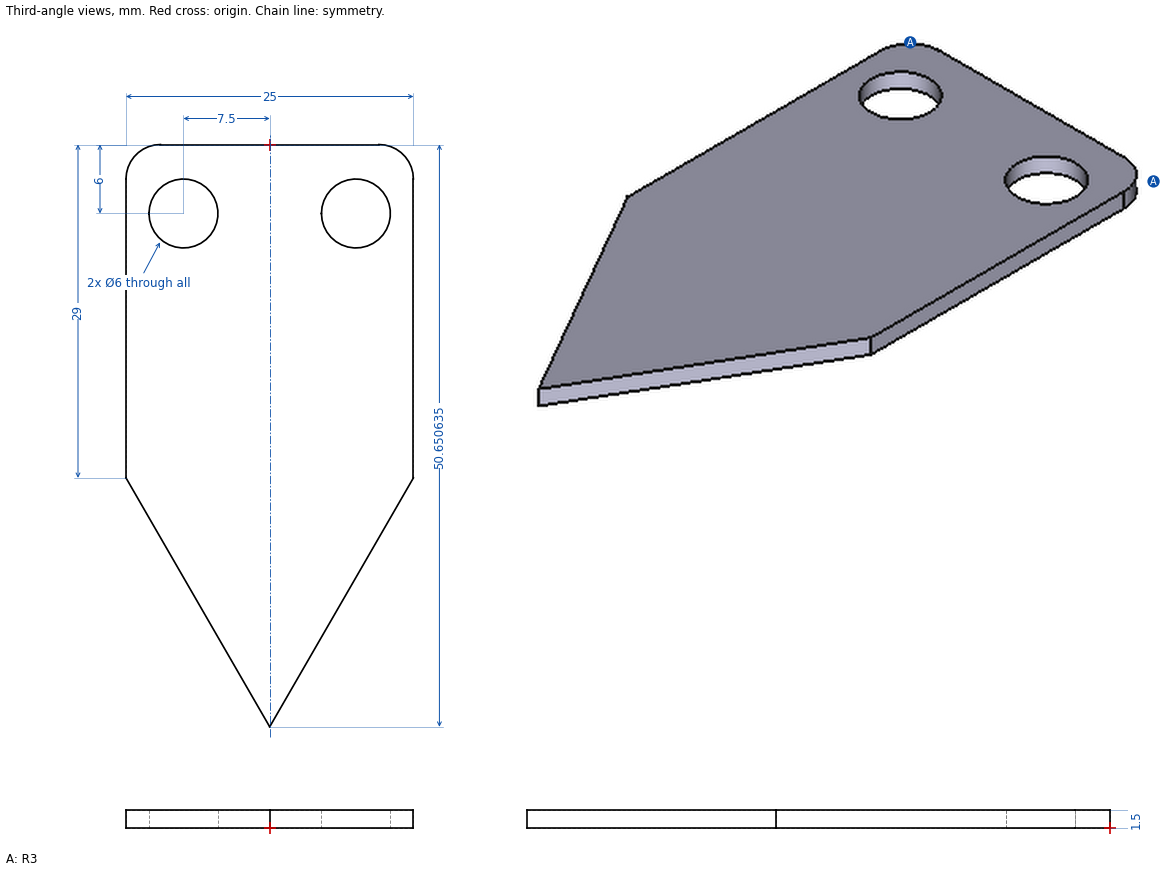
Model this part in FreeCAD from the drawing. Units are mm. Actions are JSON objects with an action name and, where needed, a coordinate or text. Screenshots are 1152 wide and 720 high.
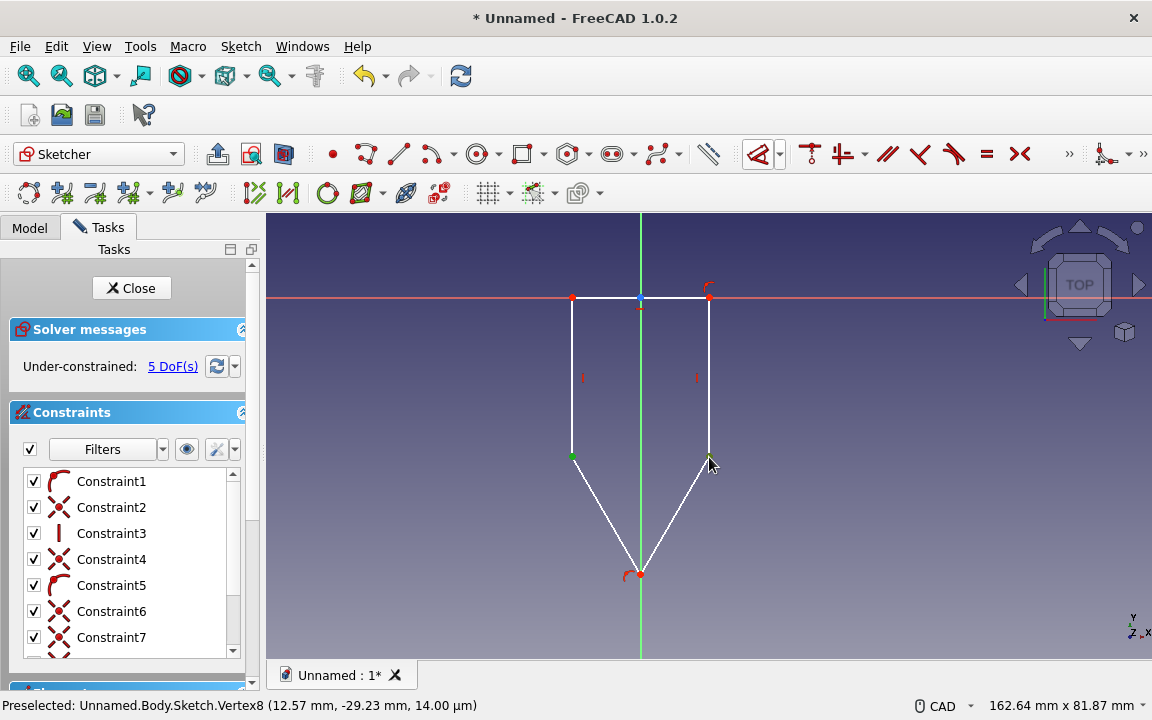
{"action": "left_click", "coordinate": [641, 492]}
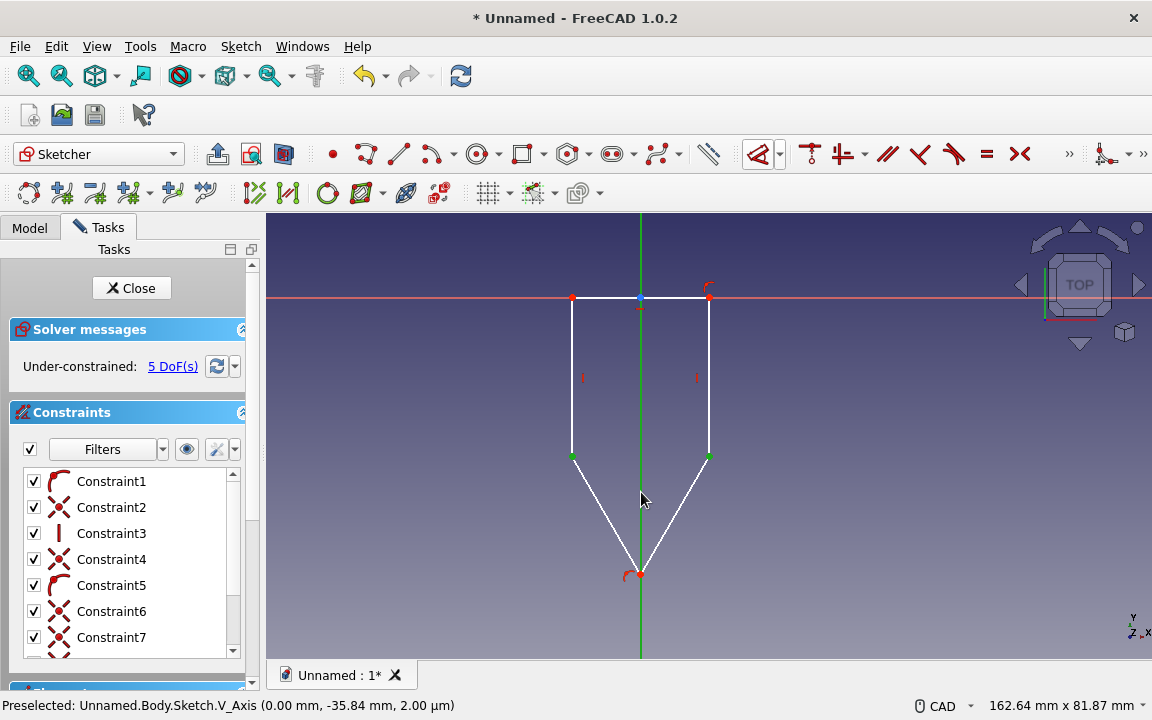
{"action": "left_click", "coordinate": [1020, 154]}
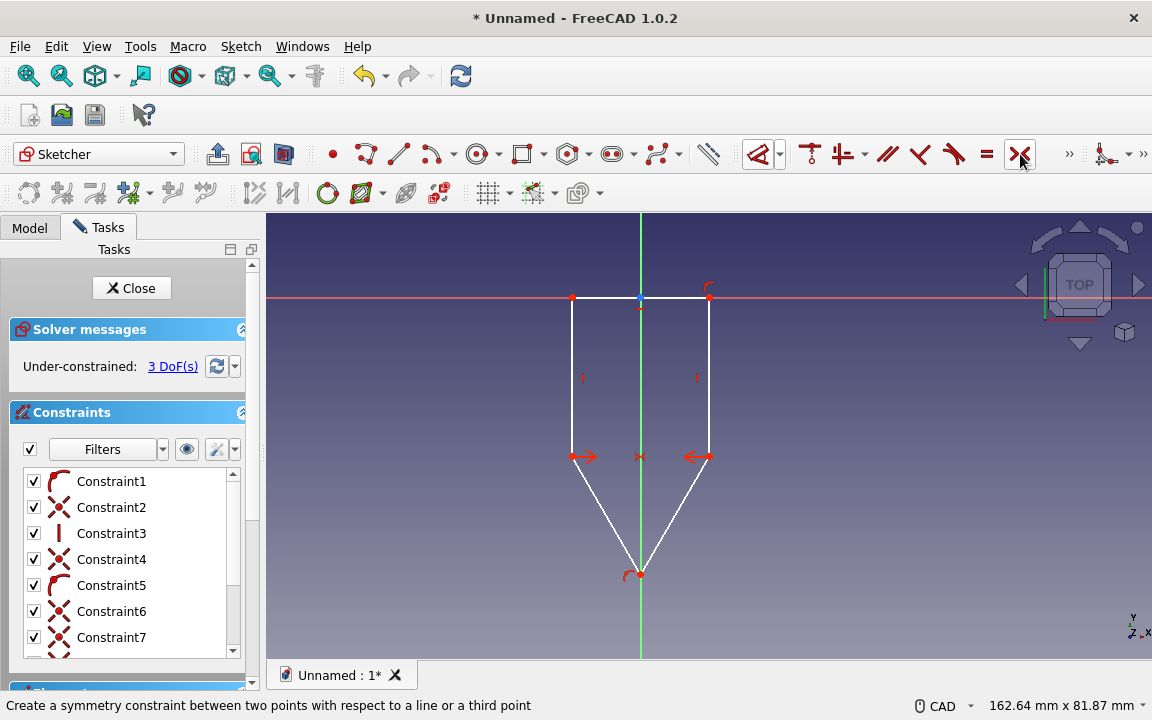
{"action": "left_click", "coordinate": [758, 154]}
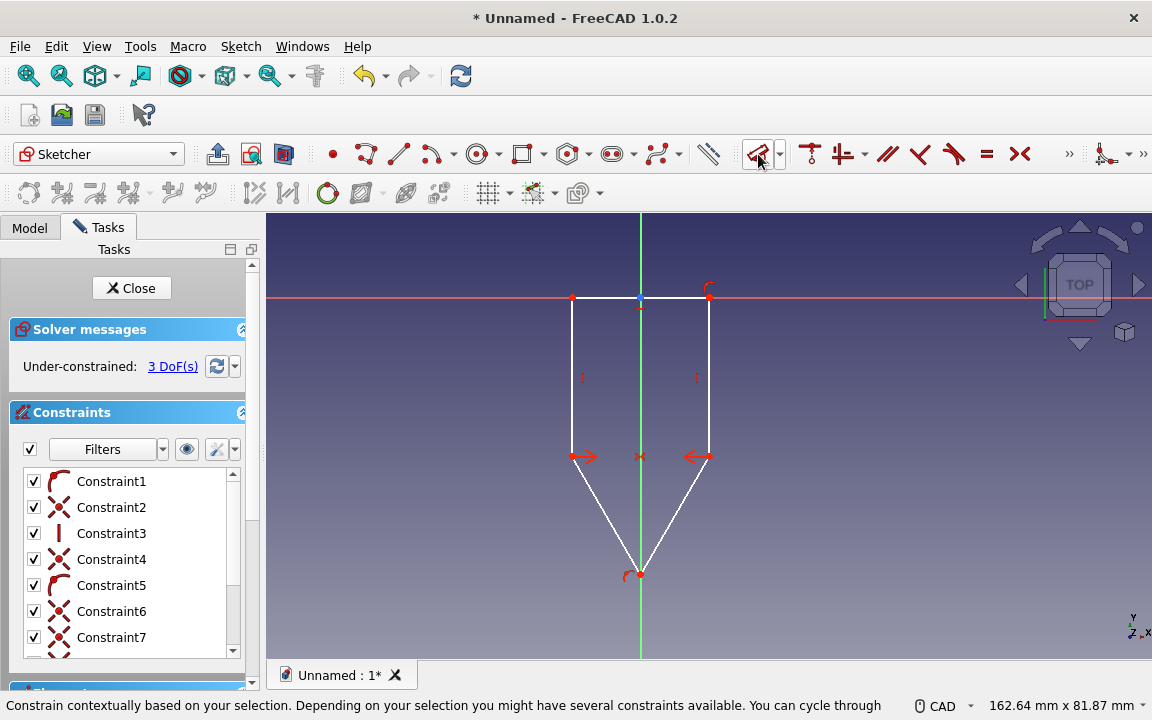
{"action": "left_click", "coordinate": [668, 298]}
{"action": "left_click", "coordinate": [609, 264]}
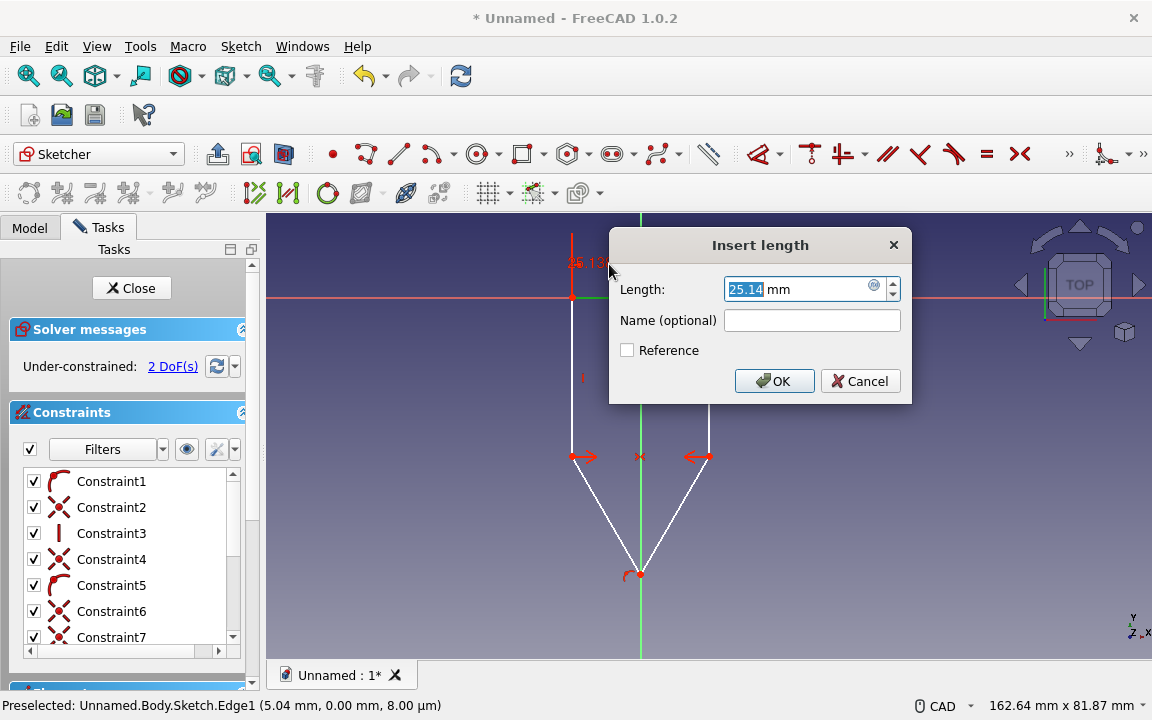
{"action": "type", "text": "25"}
{"action": "key", "text": "Return"}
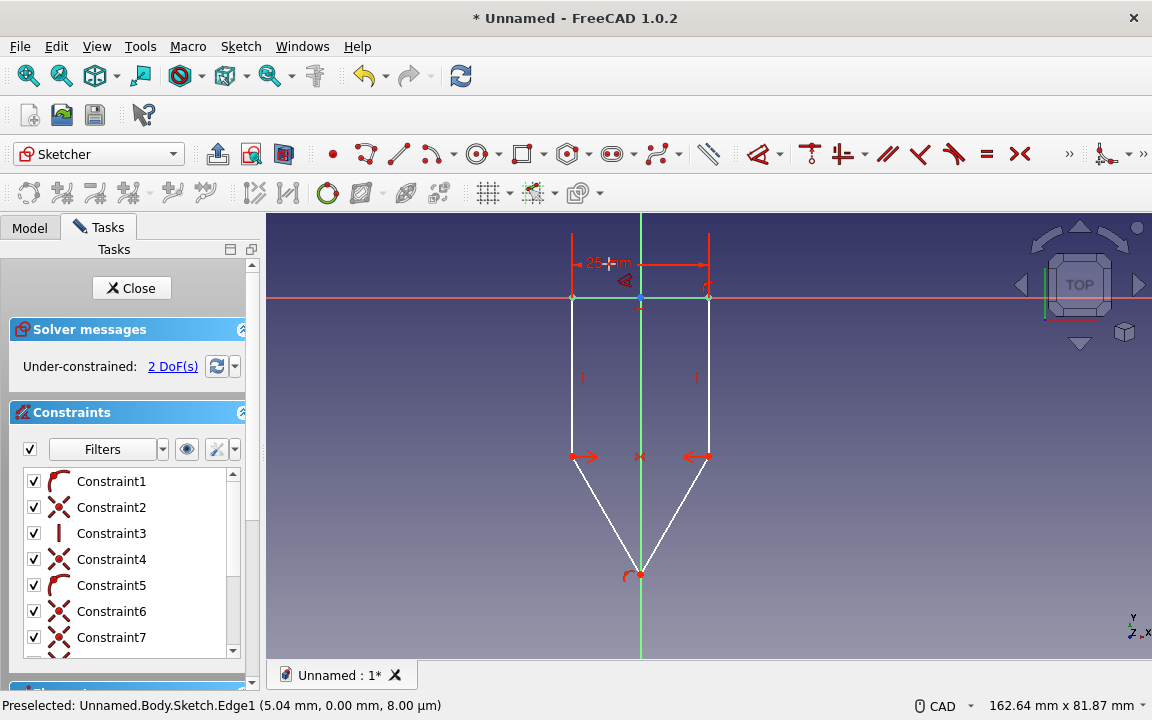
{"action": "left_click", "coordinate": [572, 346]}
{"action": "left_click", "coordinate": [538, 377]}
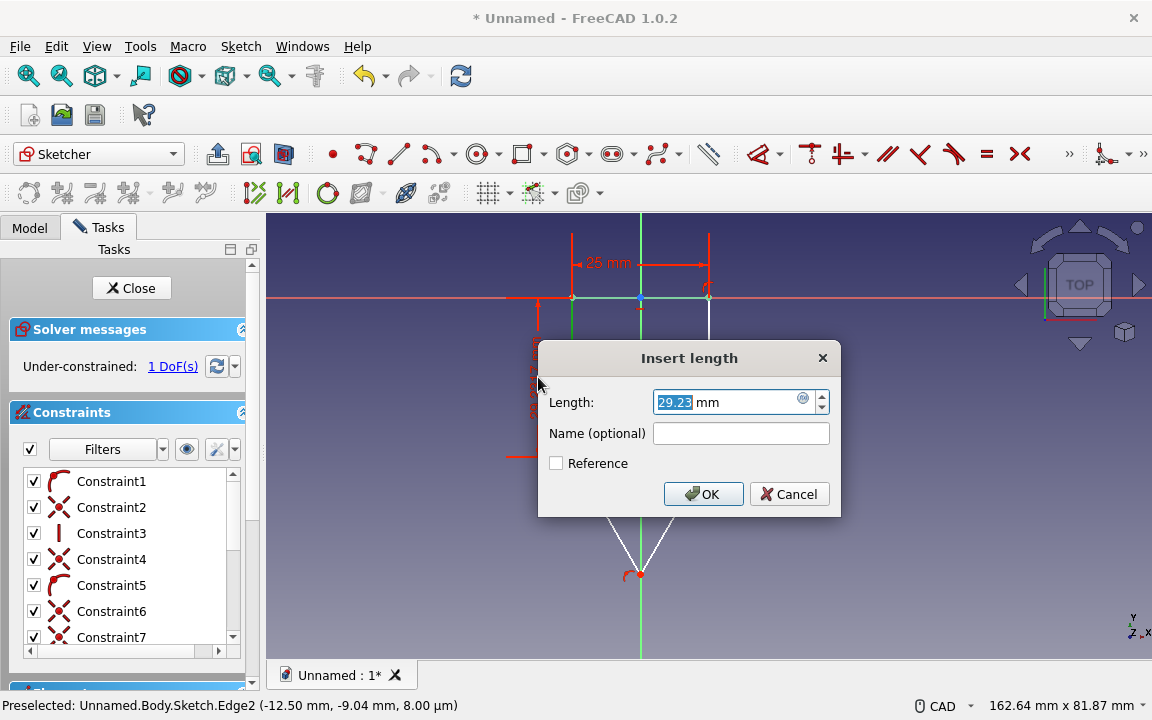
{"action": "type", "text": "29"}
{"action": "key", "text": "Return"}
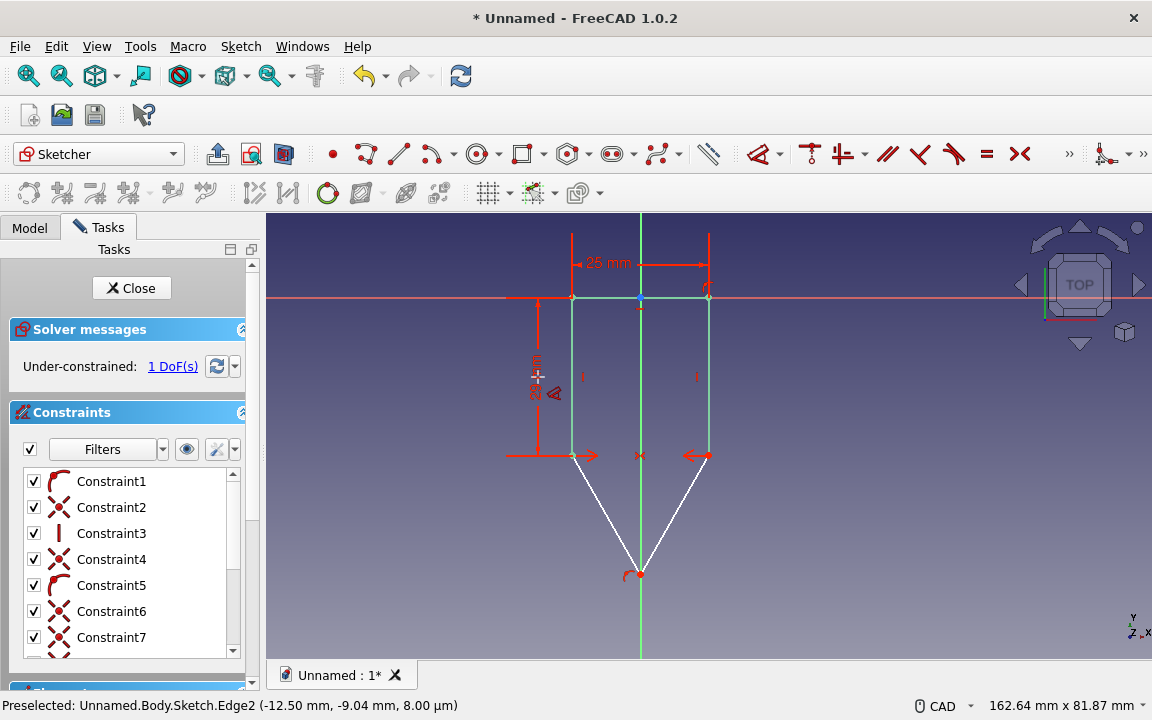
{"action": "left_click", "coordinate": [641, 575]}
{"action": "left_click", "coordinate": [675, 436]}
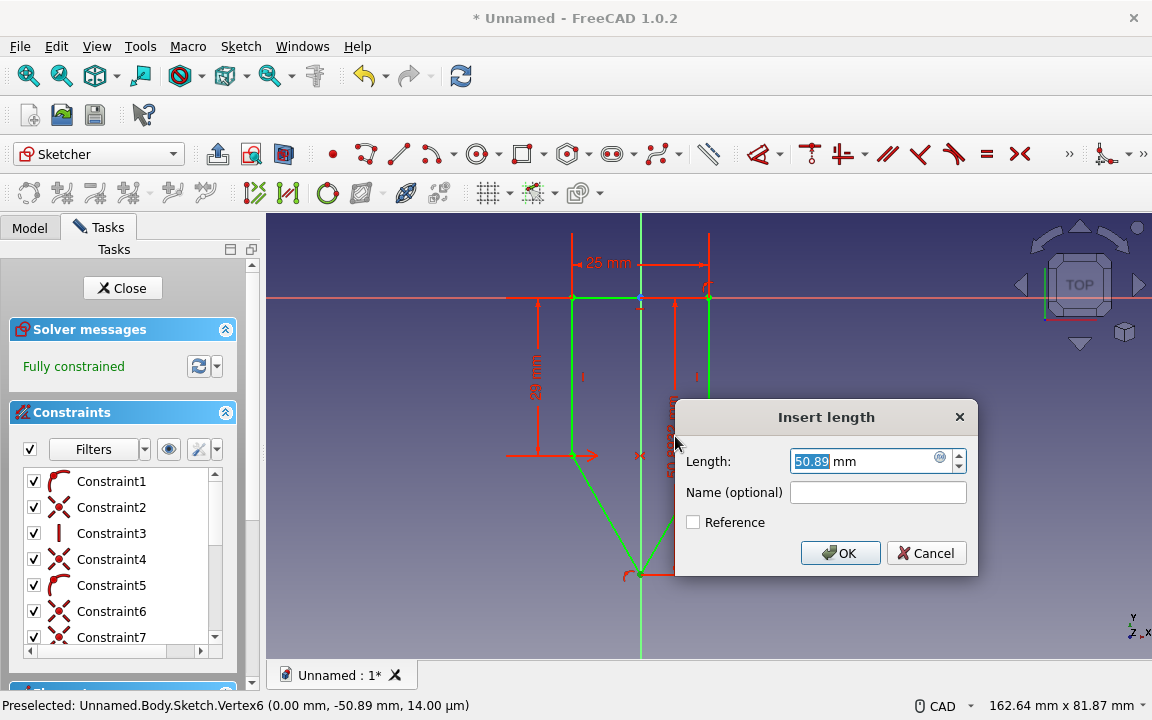
{"action": "type", "text": "50.650635"}
{"action": "key", "text": "Return"}
{"action": "key", "text": "Escape"}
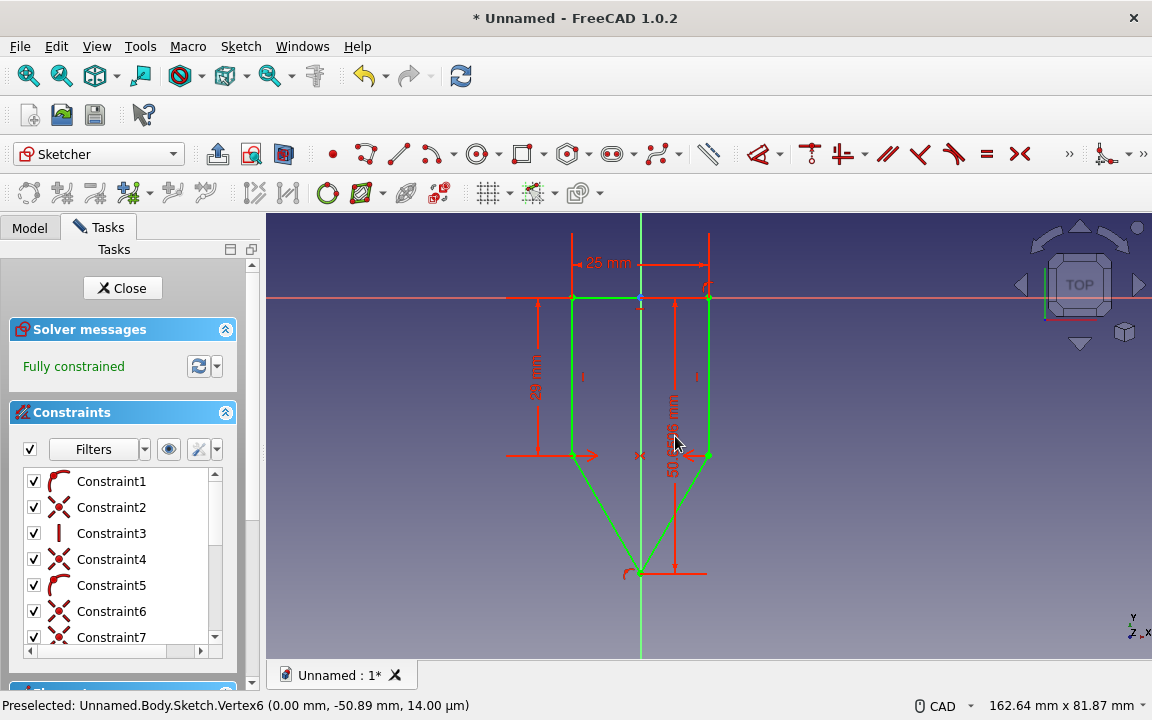
{"action": "left_click", "coordinate": [123, 288]}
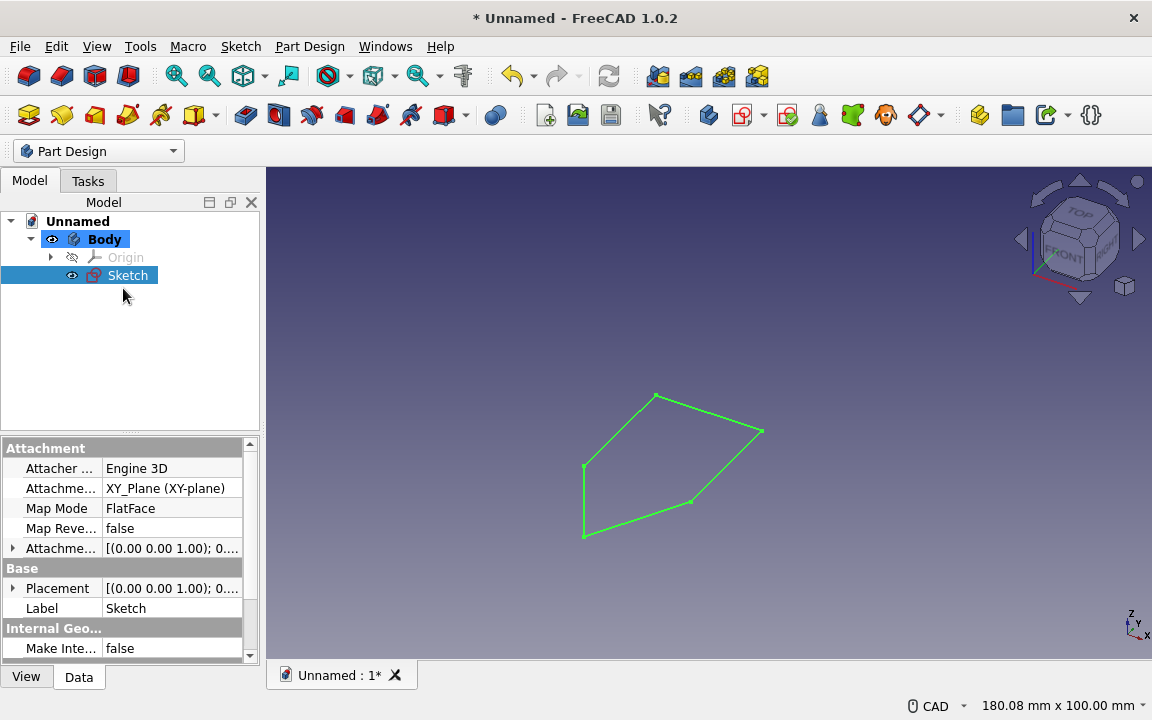
{"action": "left_click", "coordinate": [29, 116]}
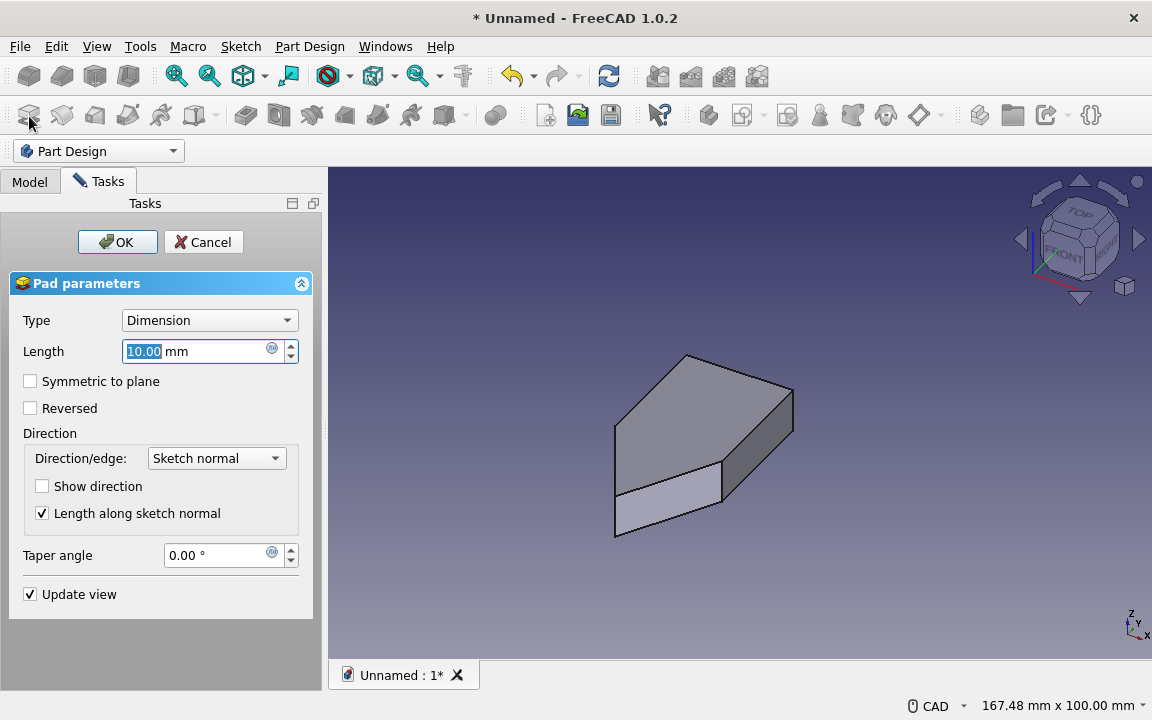
{"action": "type", "text": "1.5"}
{"action": "key", "text": "Tab"}